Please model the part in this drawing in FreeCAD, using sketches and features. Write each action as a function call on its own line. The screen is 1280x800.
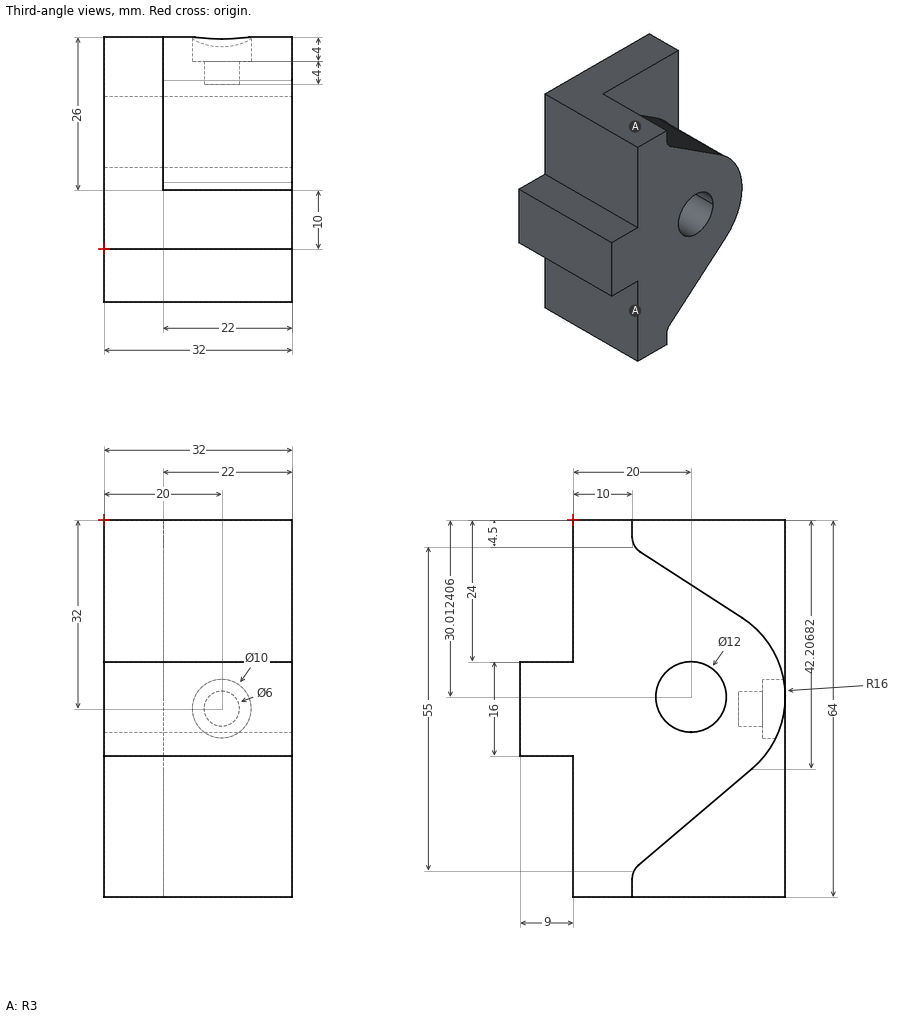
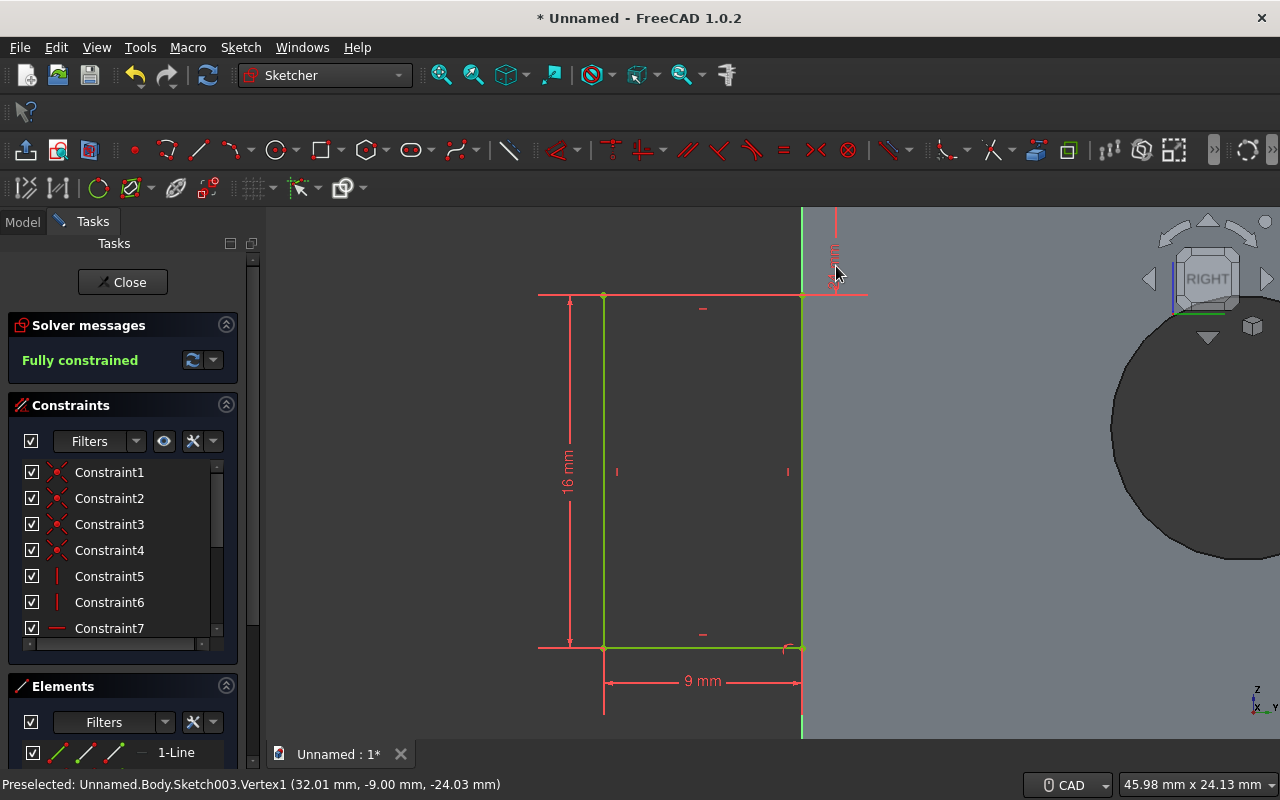
click(123, 282)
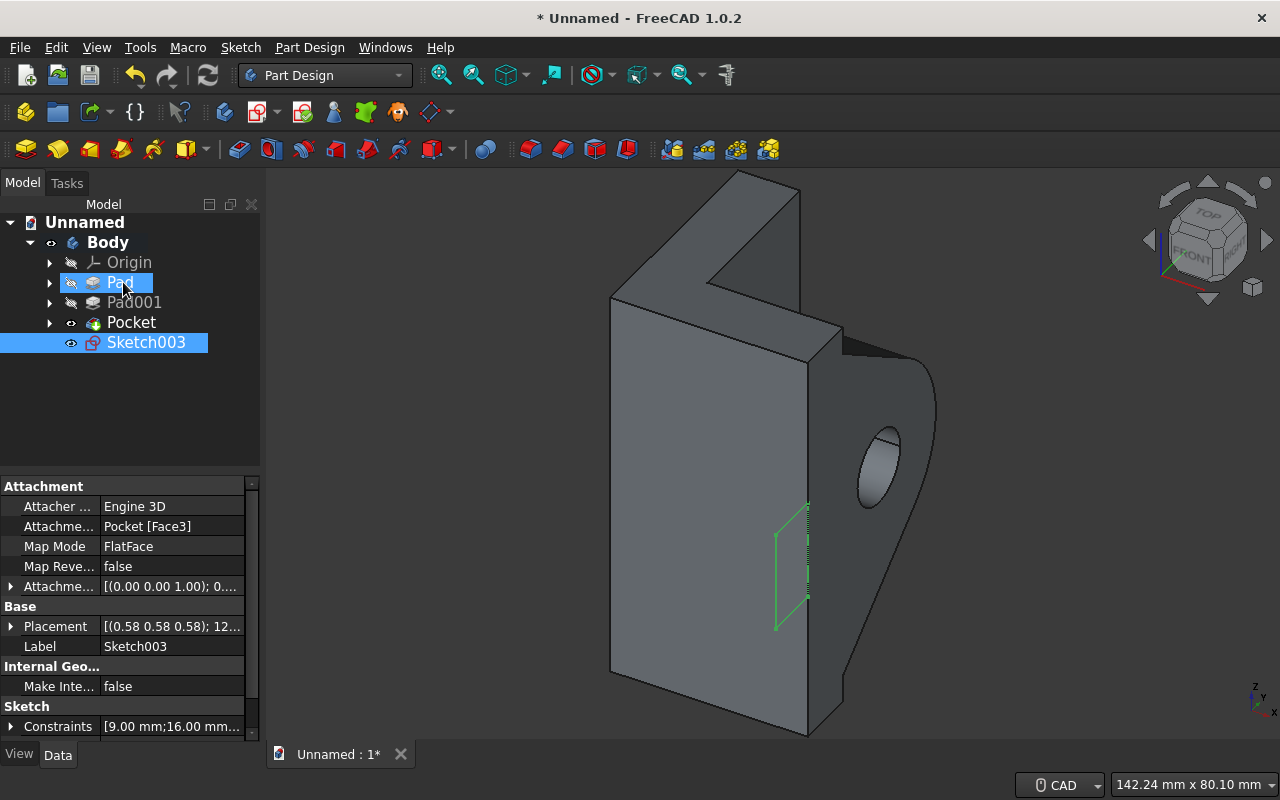
click(26, 150)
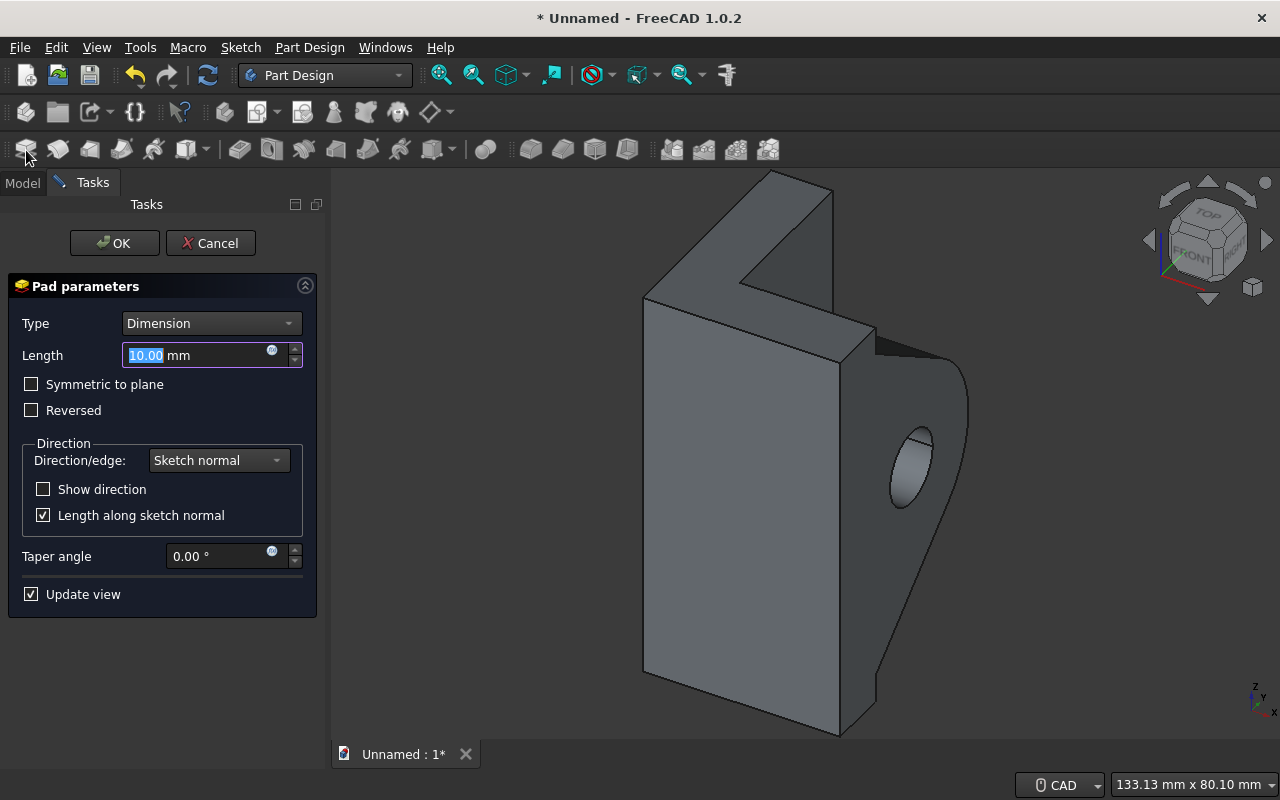
text(32)
key(Tab)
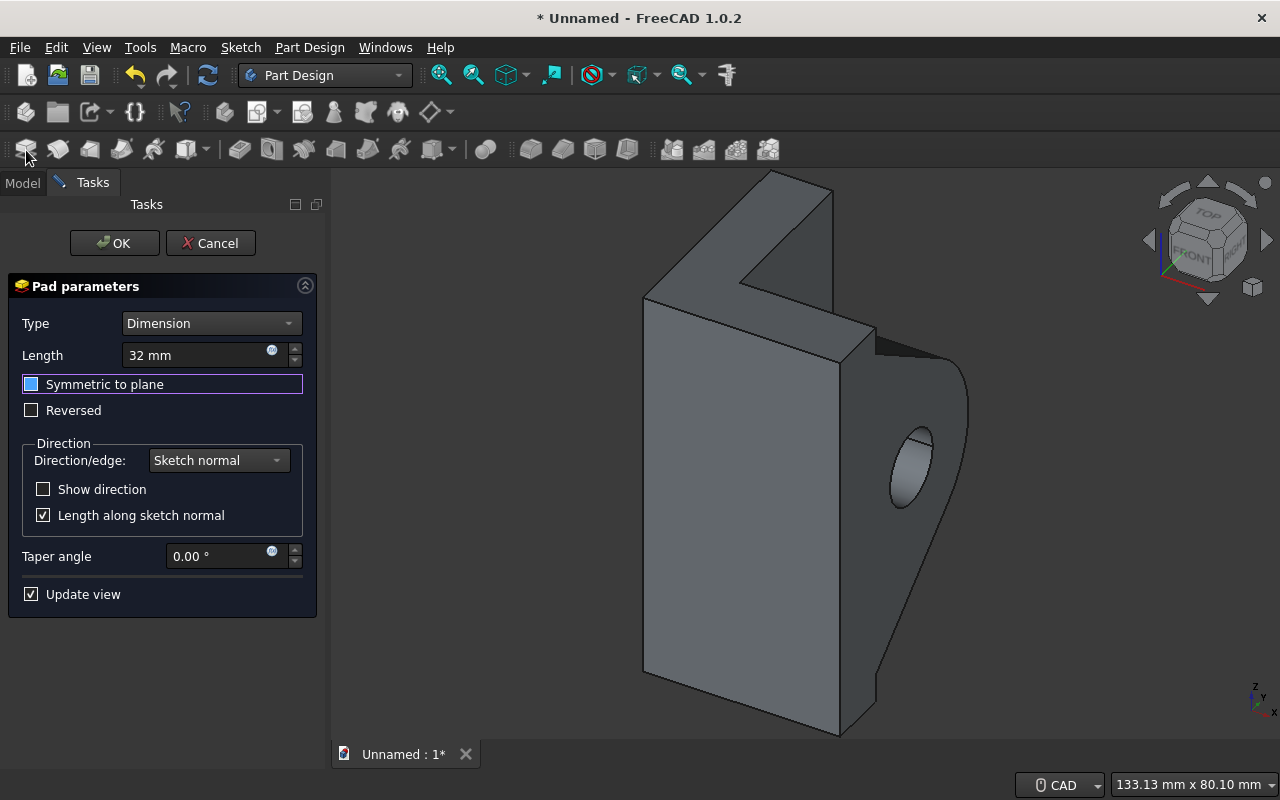
click(30, 410)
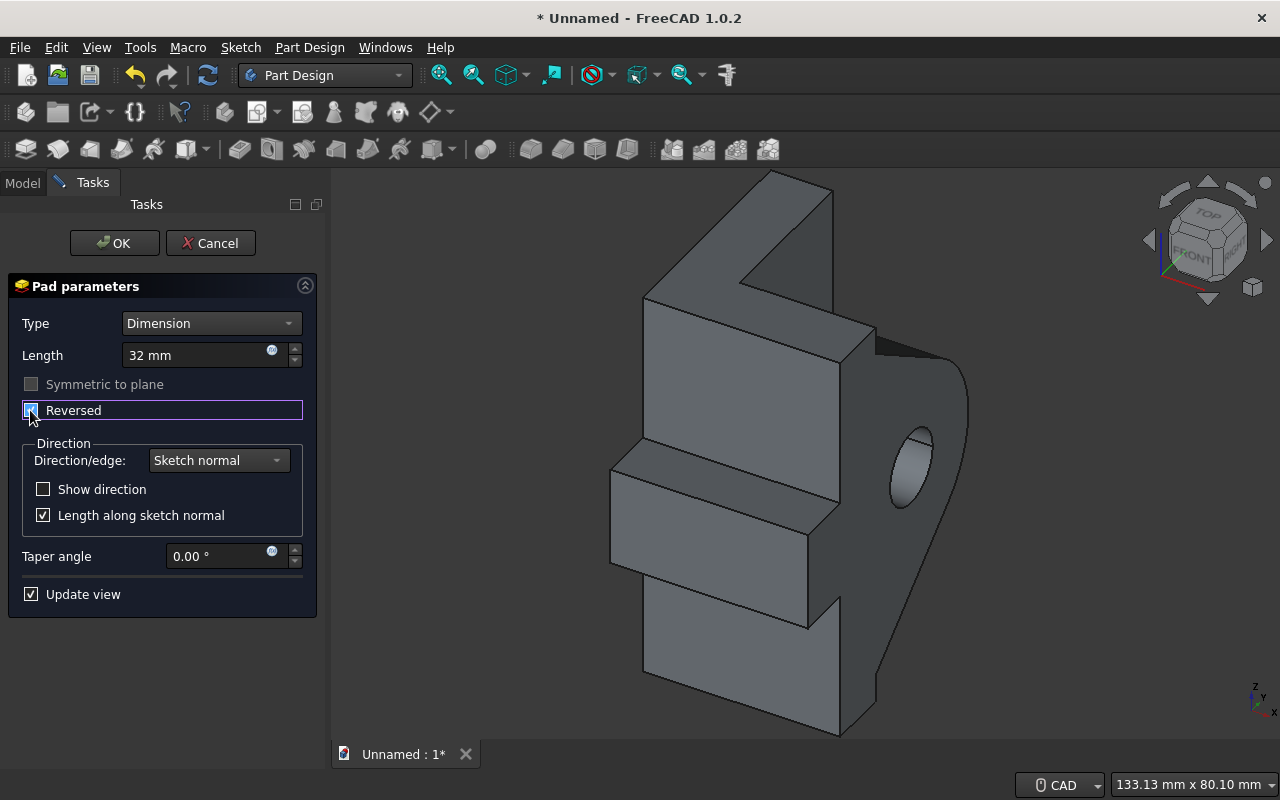
click(115, 243)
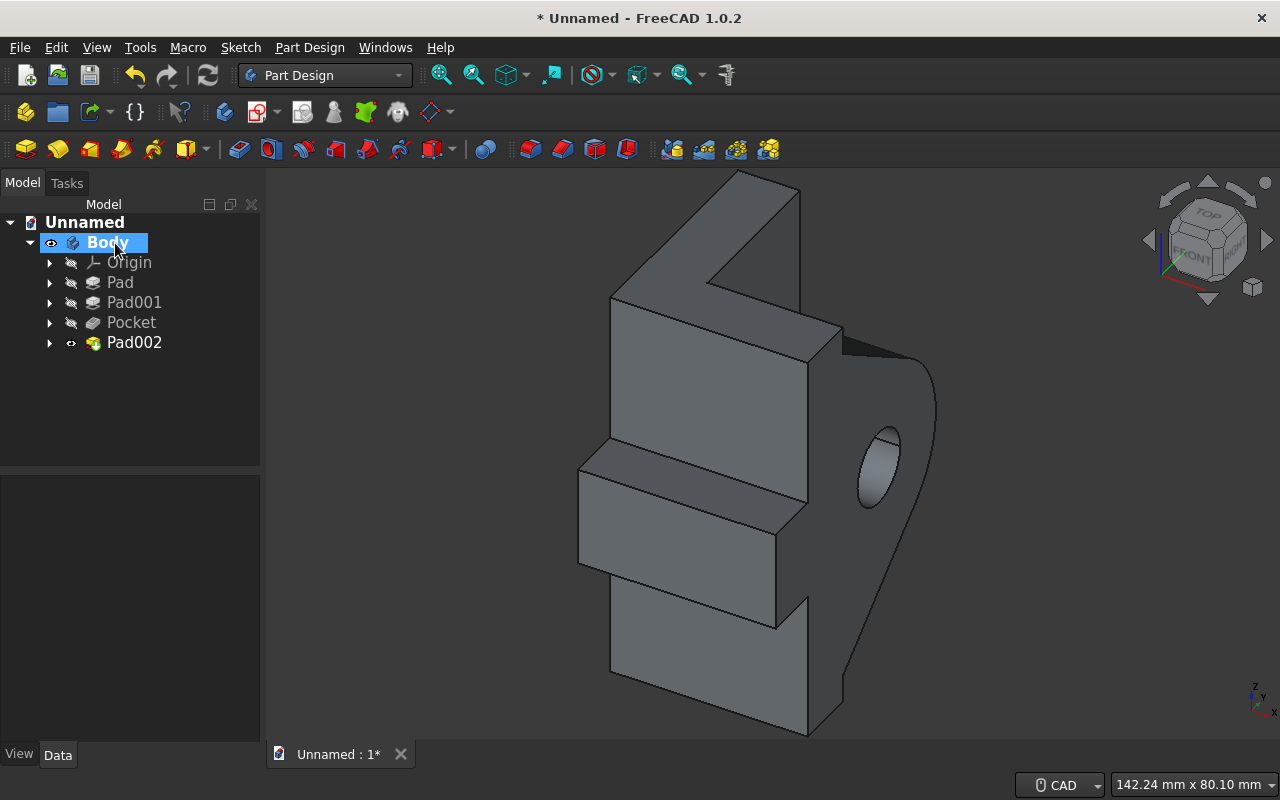
key(v)
key(f)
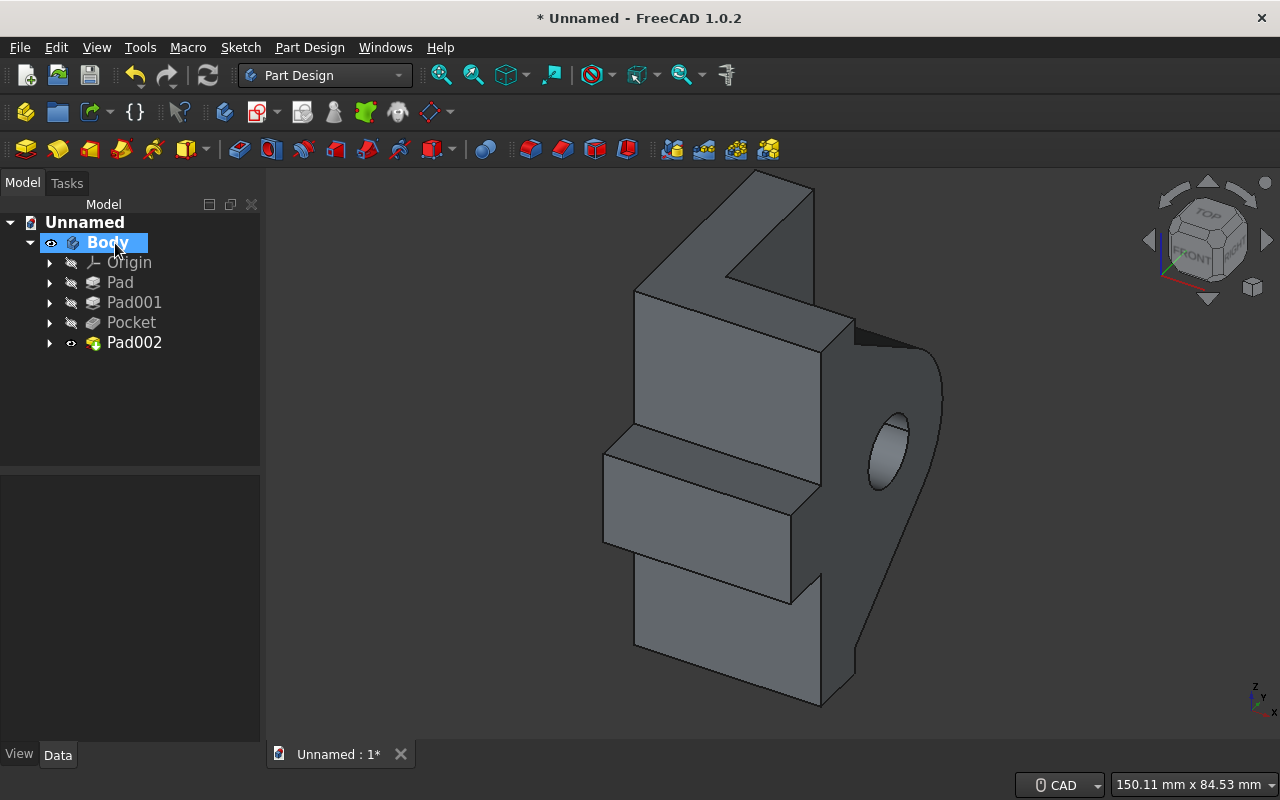
key(0)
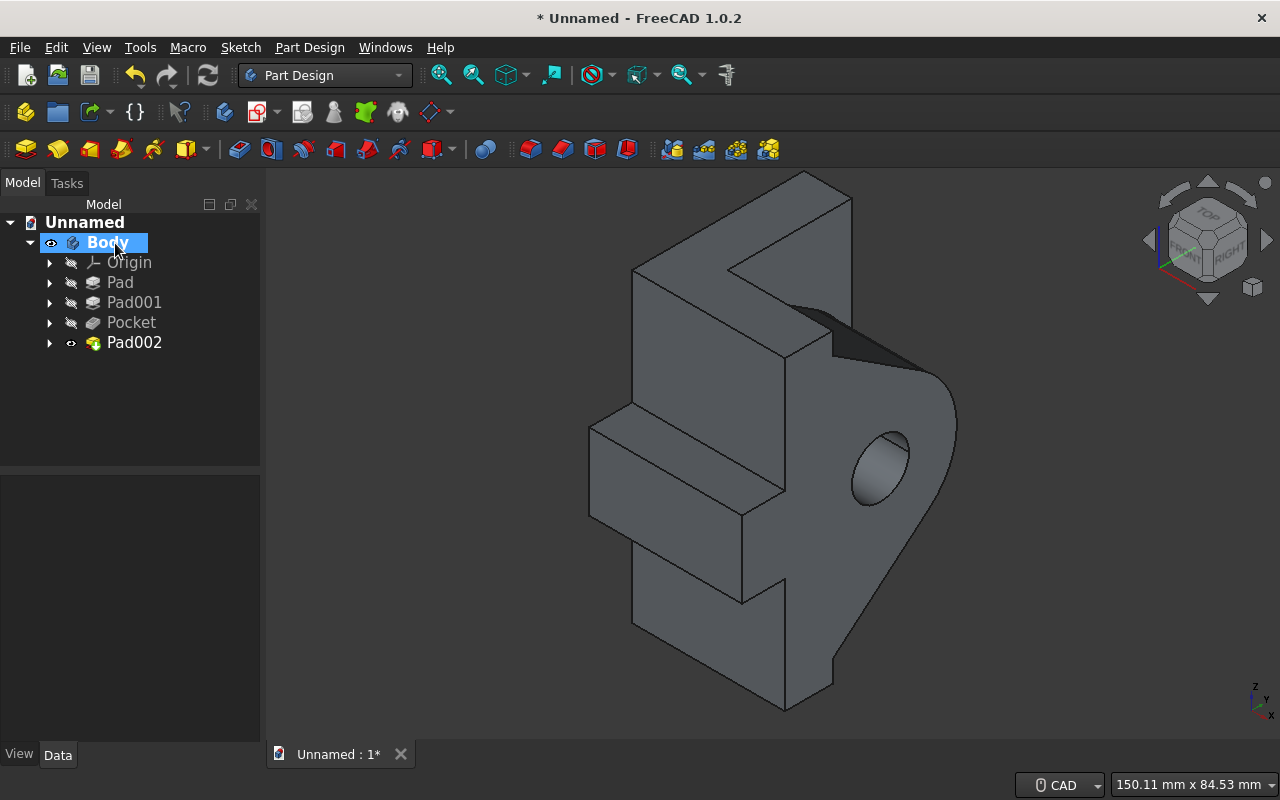
key(2)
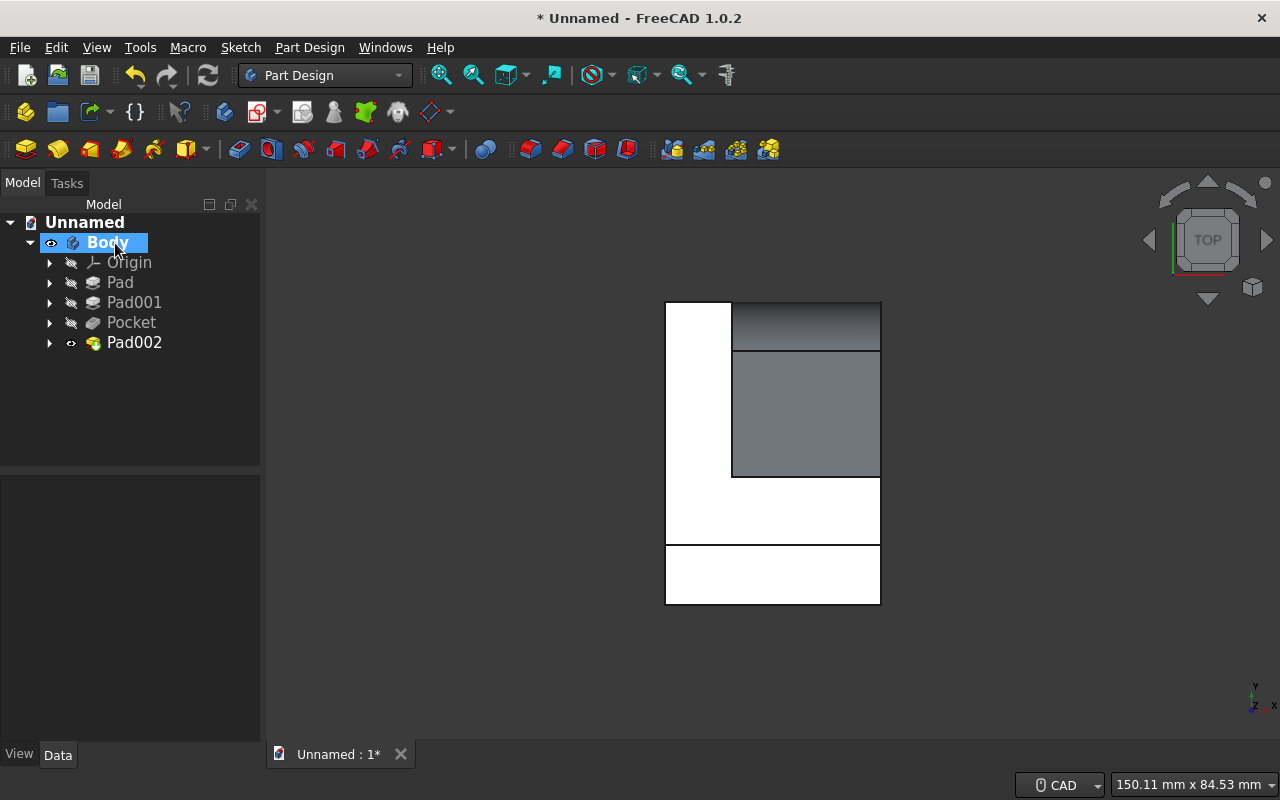
key(1)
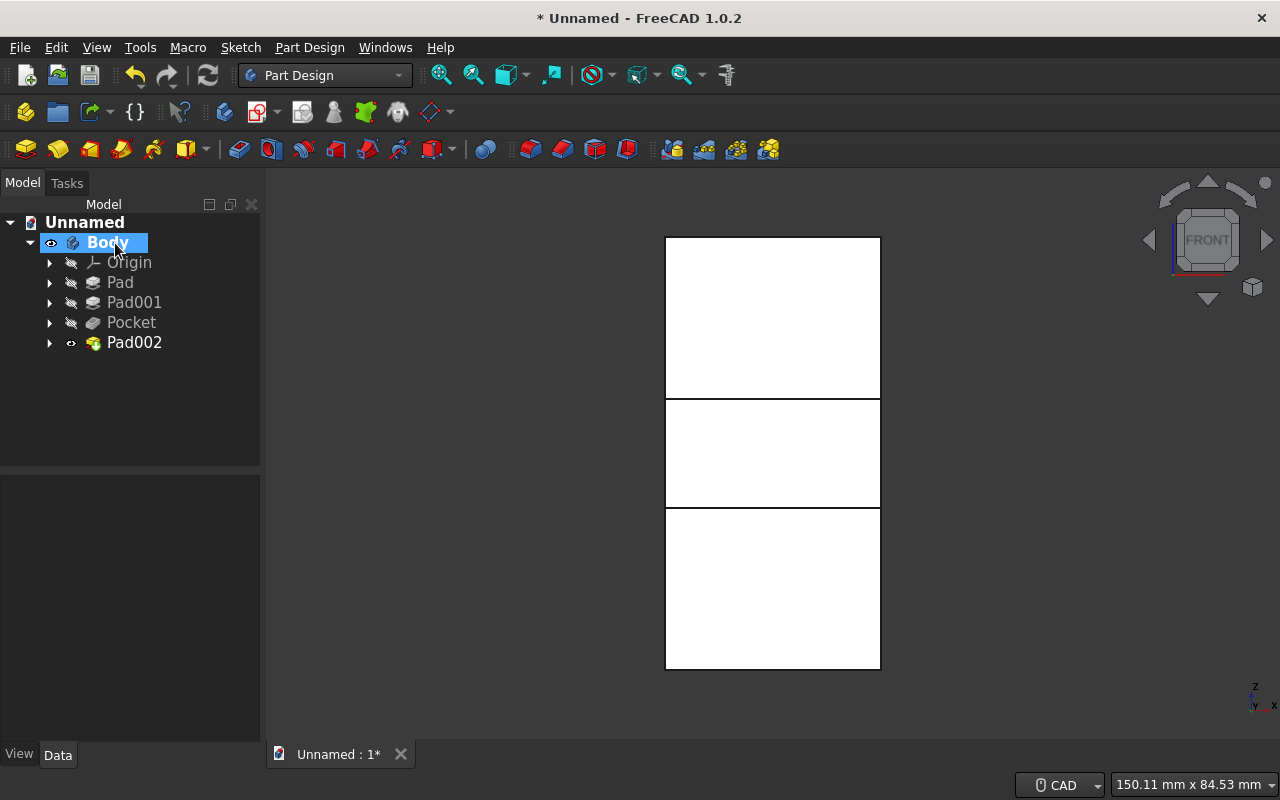
key(3)